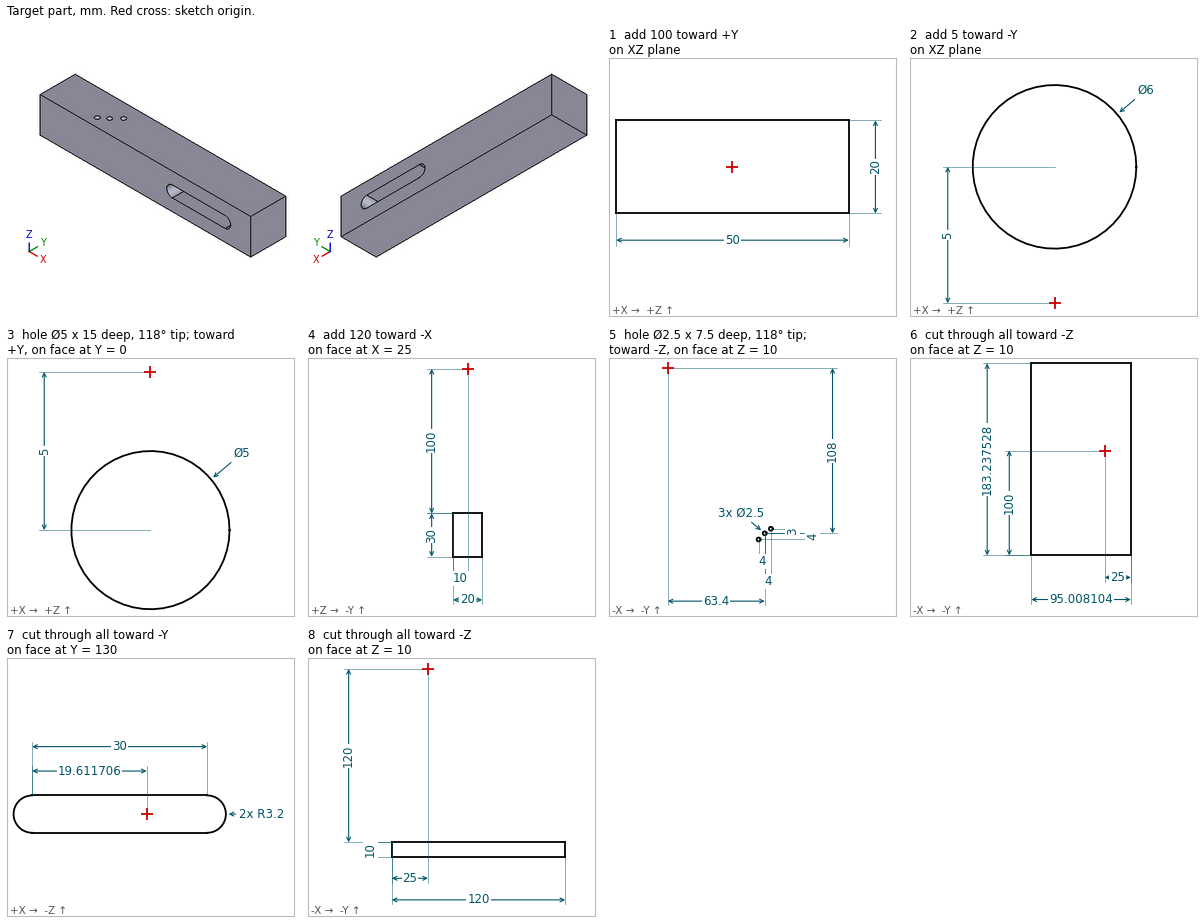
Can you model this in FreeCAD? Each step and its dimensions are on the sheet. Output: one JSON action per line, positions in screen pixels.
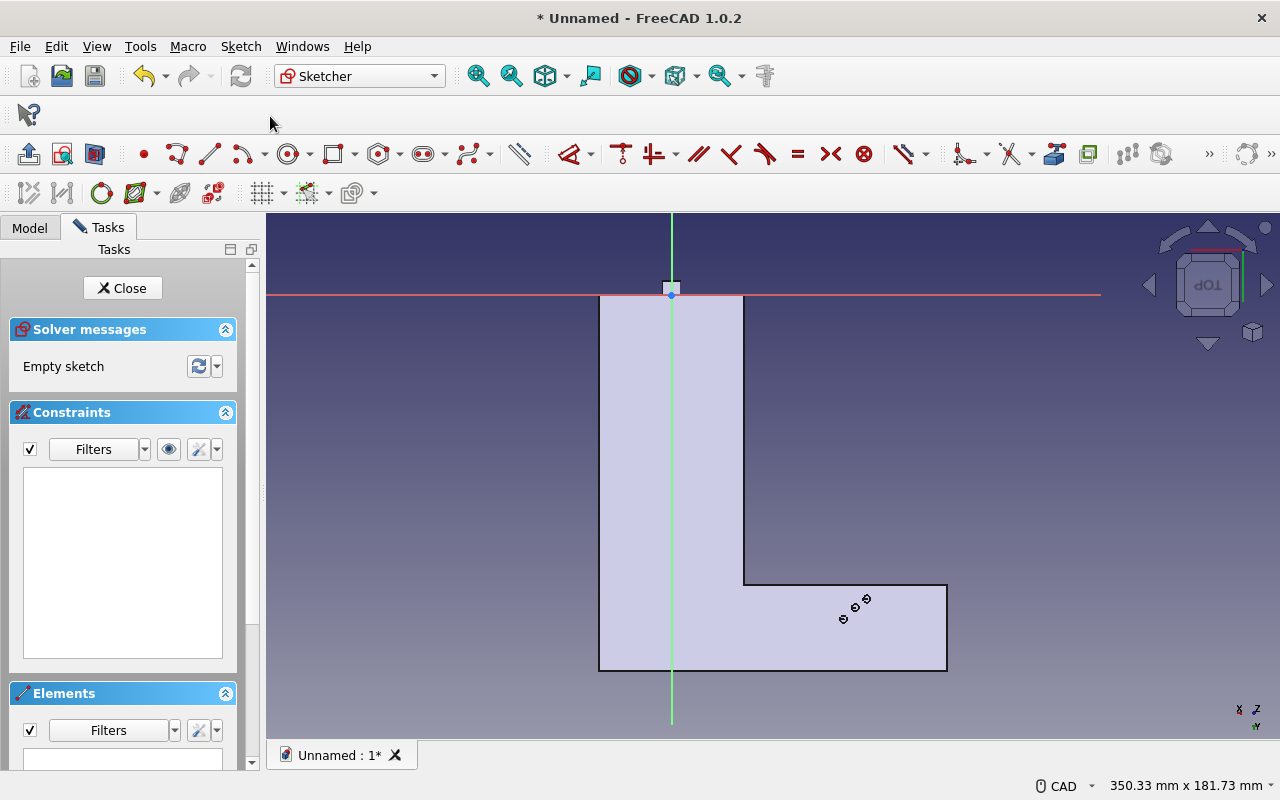
{"action": "scroll", "coordinate": [904, 711], "scroll_direction": "down", "scroll_amount": 2}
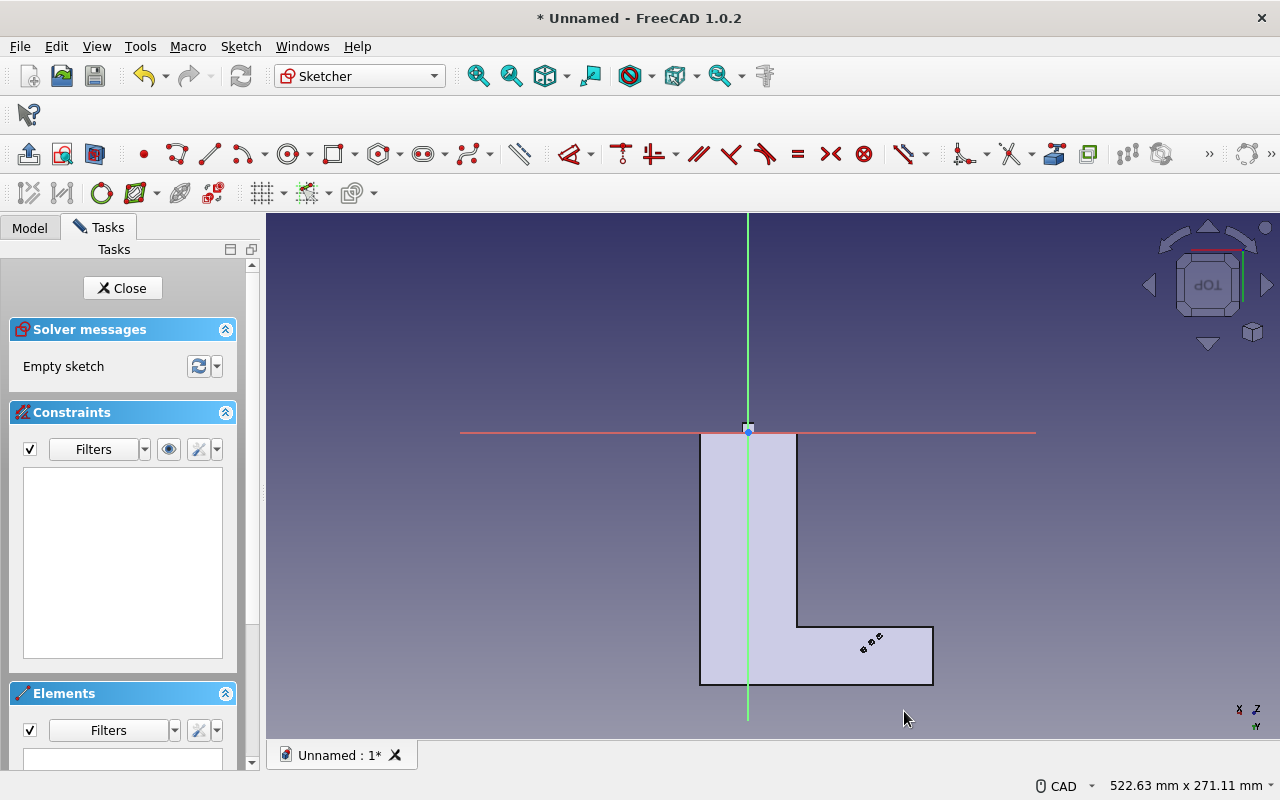
{"action": "left_click", "coordinate": [332, 154]}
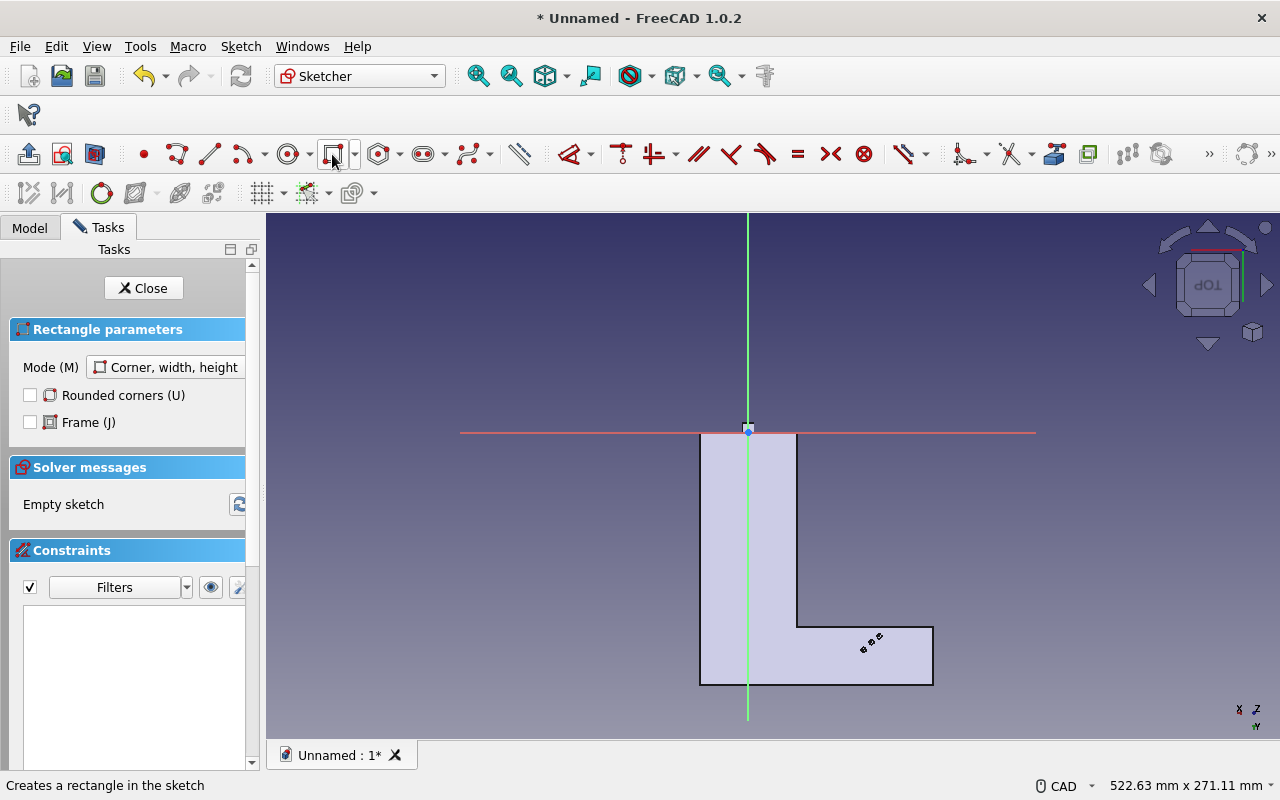
{"action": "left_click", "coordinate": [613, 271]}
{"action": "left_click", "coordinate": [797, 627]}
{"action": "key", "text": "Escape"}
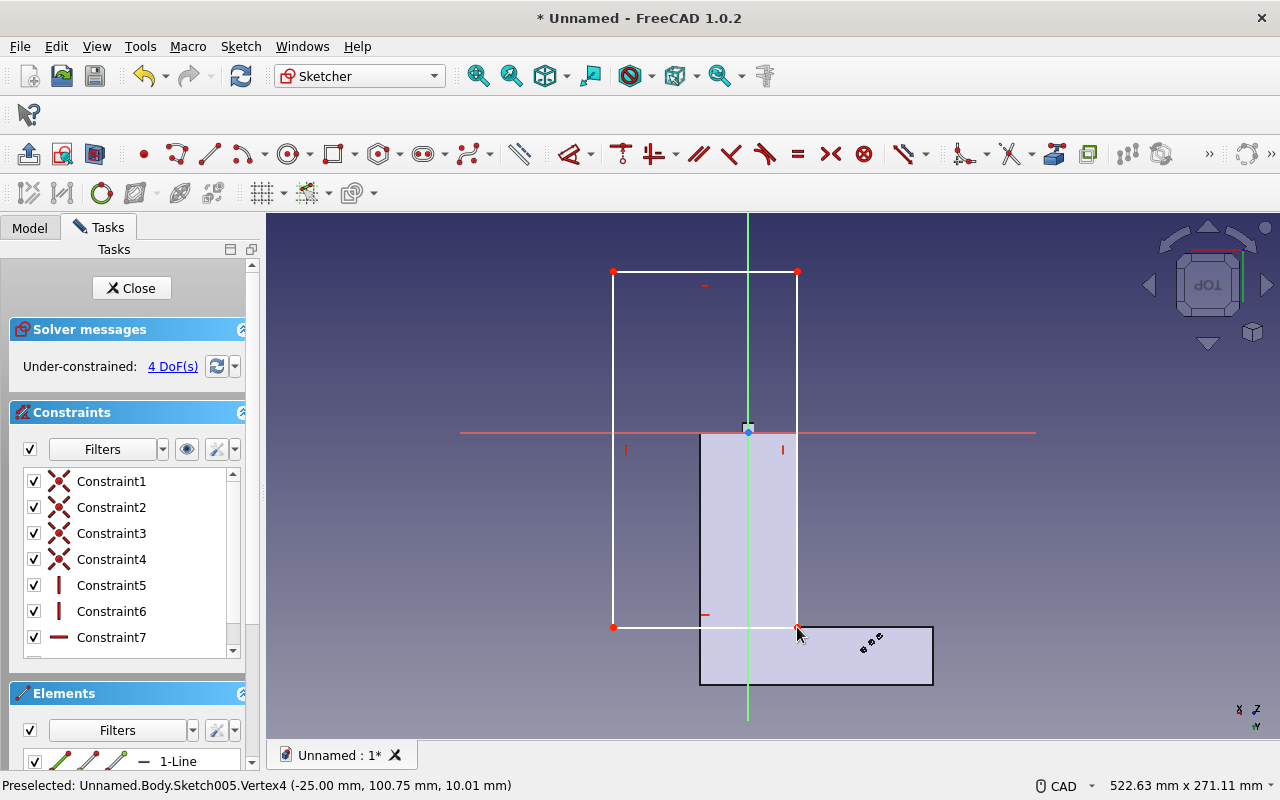
{"action": "left_click", "coordinate": [568, 154]}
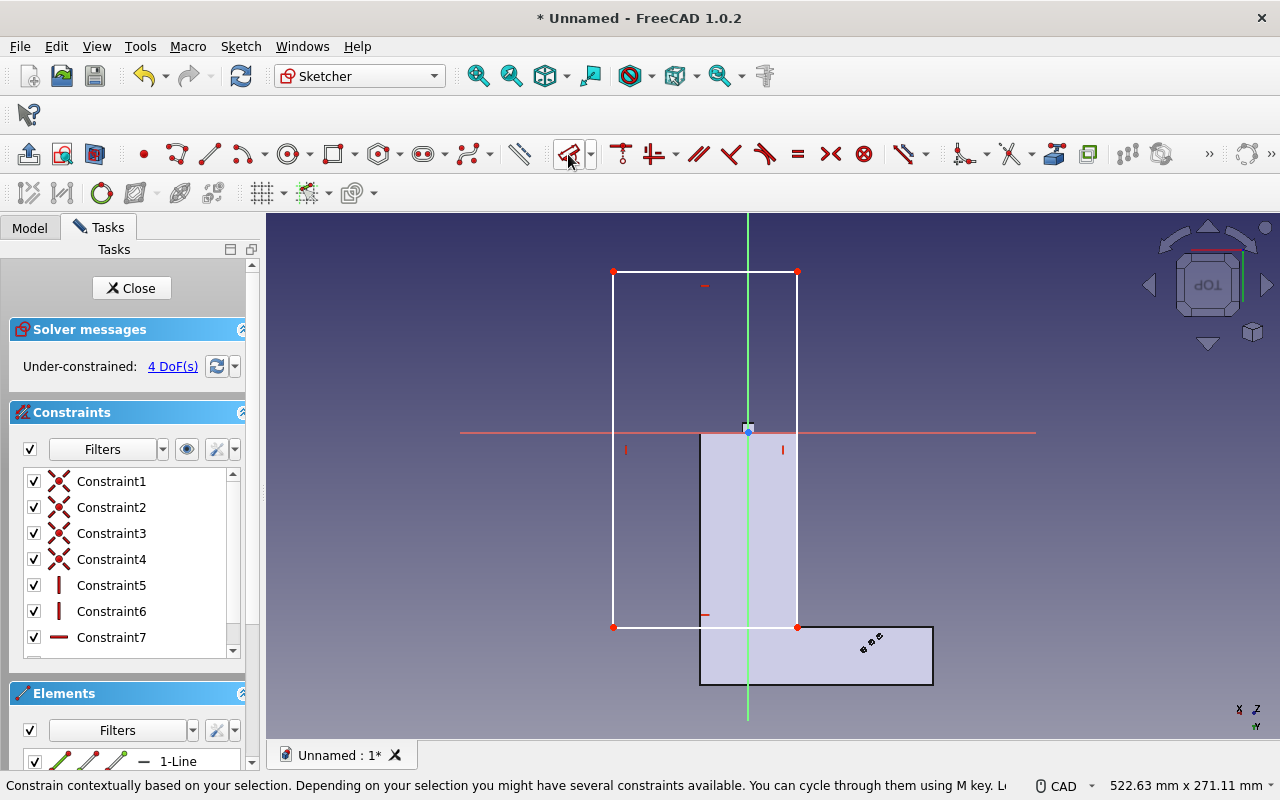
{"action": "left_click", "coordinate": [797, 628]}
{"action": "left_click", "coordinate": [773, 662]}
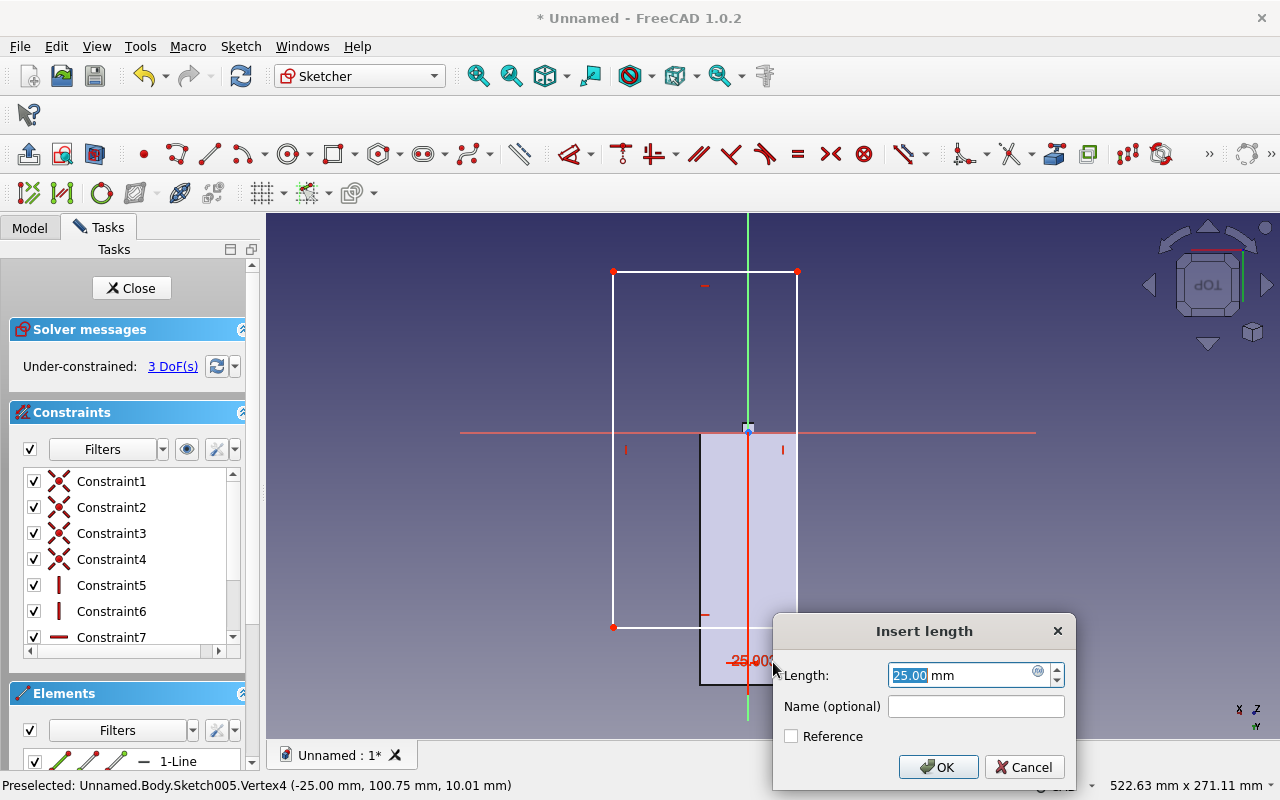
{"action": "type", "text": "25"}
{"action": "key", "text": "Return"}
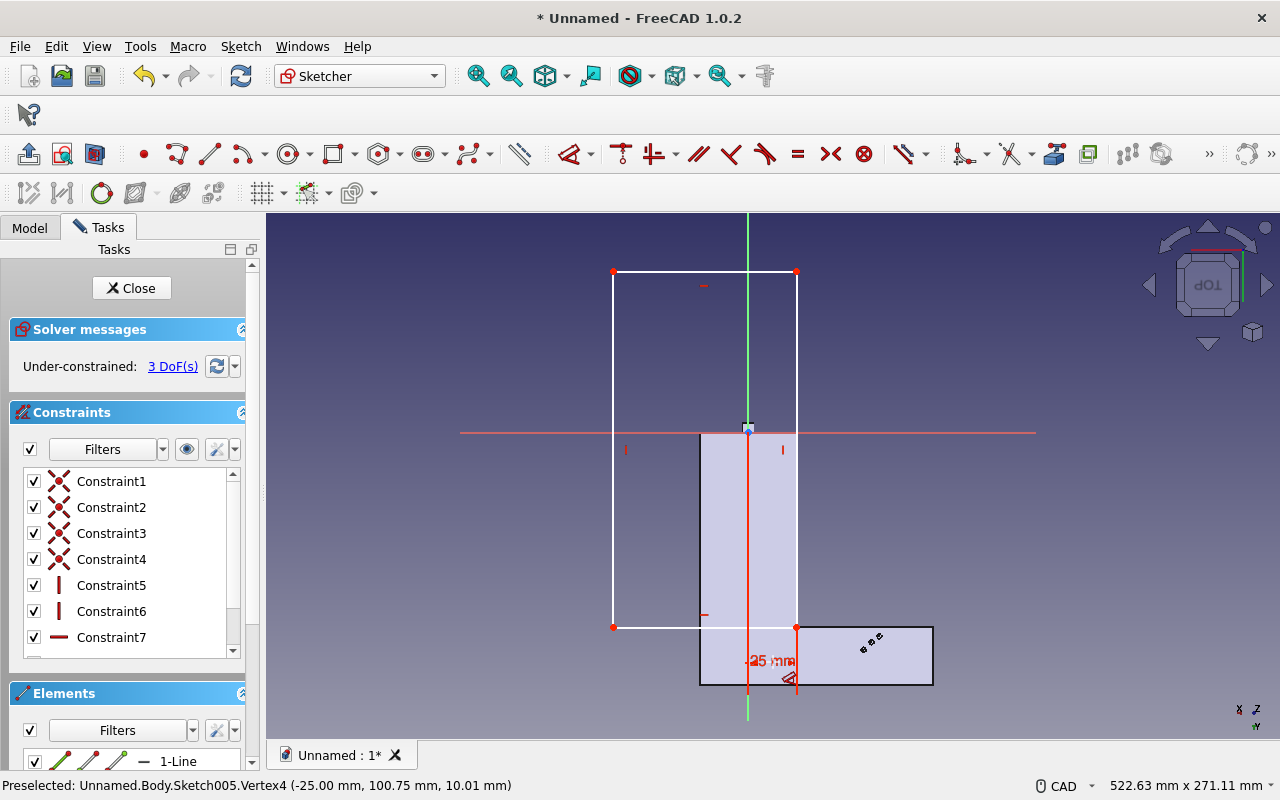
{"action": "left_click", "coordinate": [613, 628]}
{"action": "left_click", "coordinate": [579, 530]}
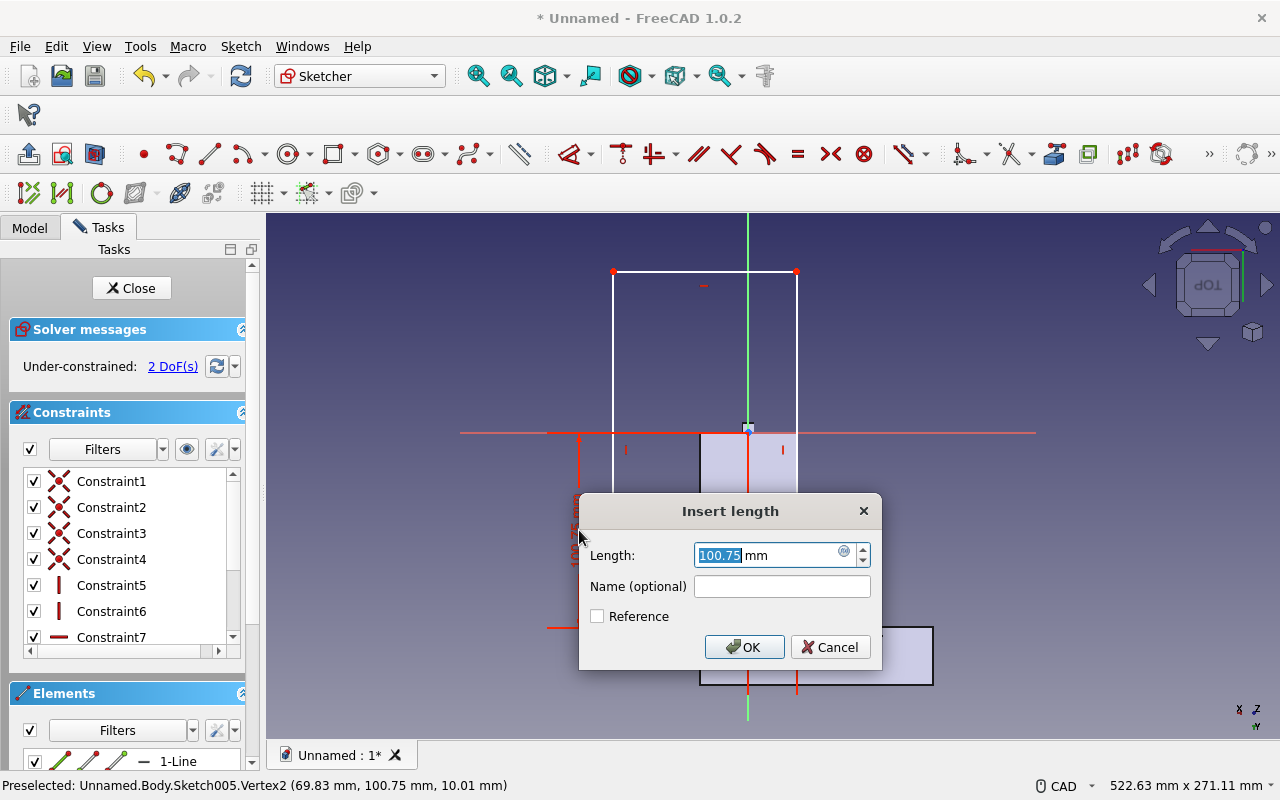
{"action": "type", "text": "100"}
{"action": "key", "text": "Return"}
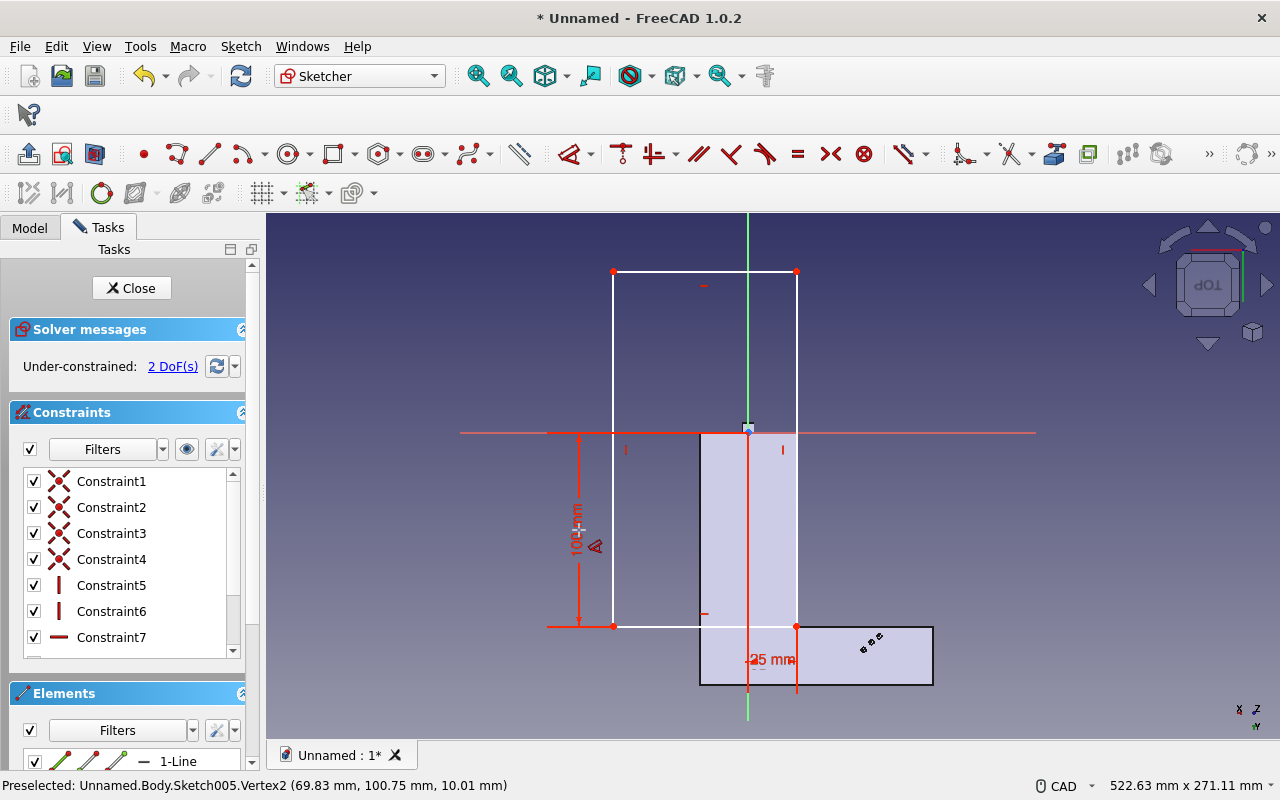
{"action": "left_click", "coordinate": [668, 627]}
{"action": "left_click", "coordinate": [663, 661]}